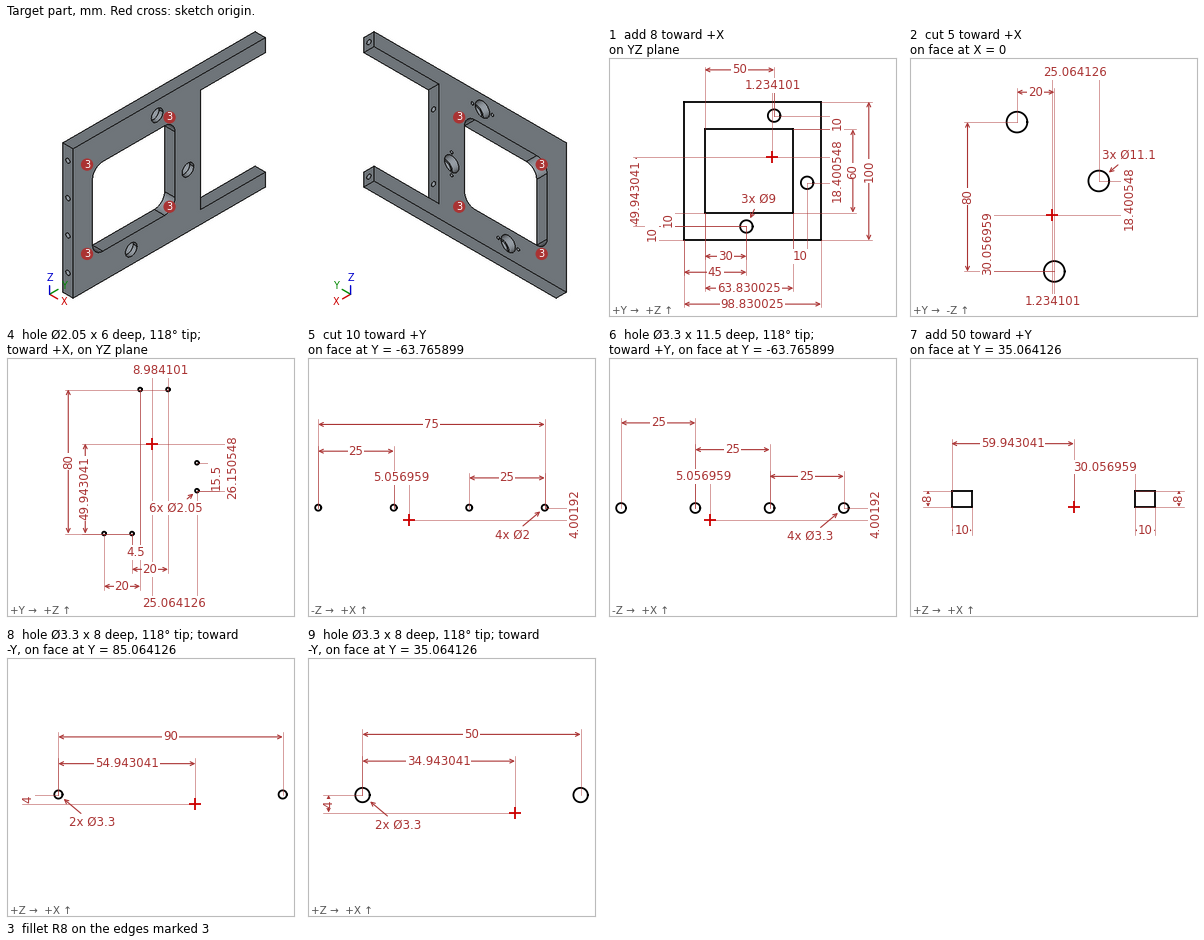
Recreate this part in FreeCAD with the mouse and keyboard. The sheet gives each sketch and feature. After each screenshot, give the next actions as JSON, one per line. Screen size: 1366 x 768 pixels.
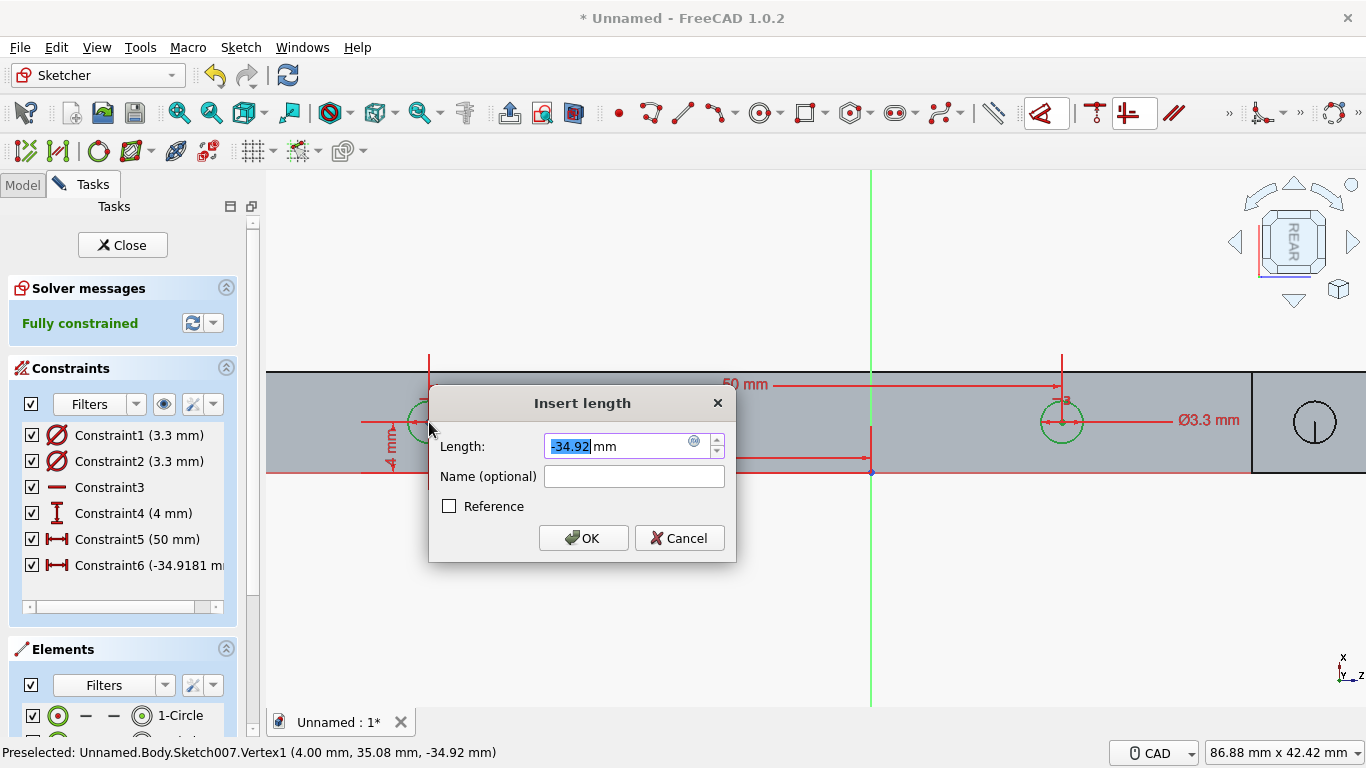
{"action": "type", "text": "-34.943041"}
{"action": "key", "text": "Return"}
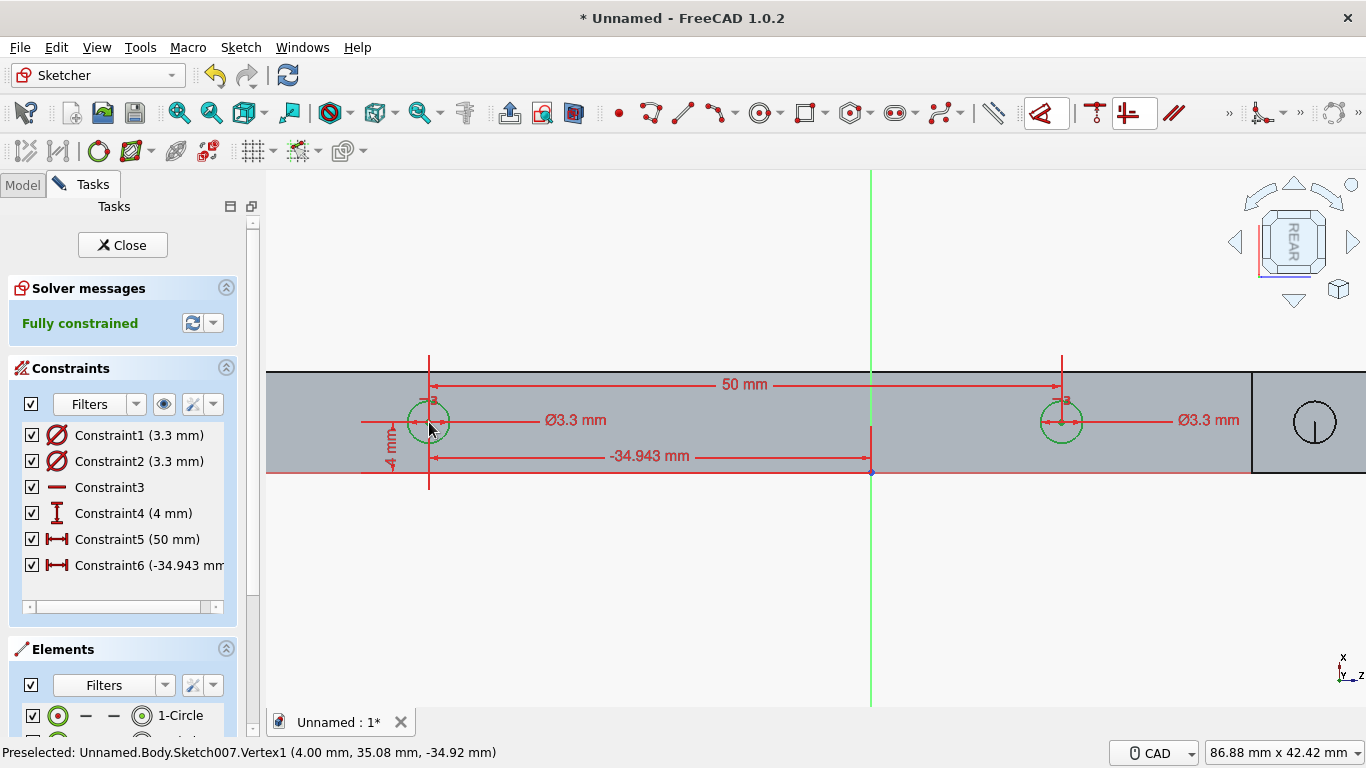
{"action": "left_click", "coordinate": [123, 245]}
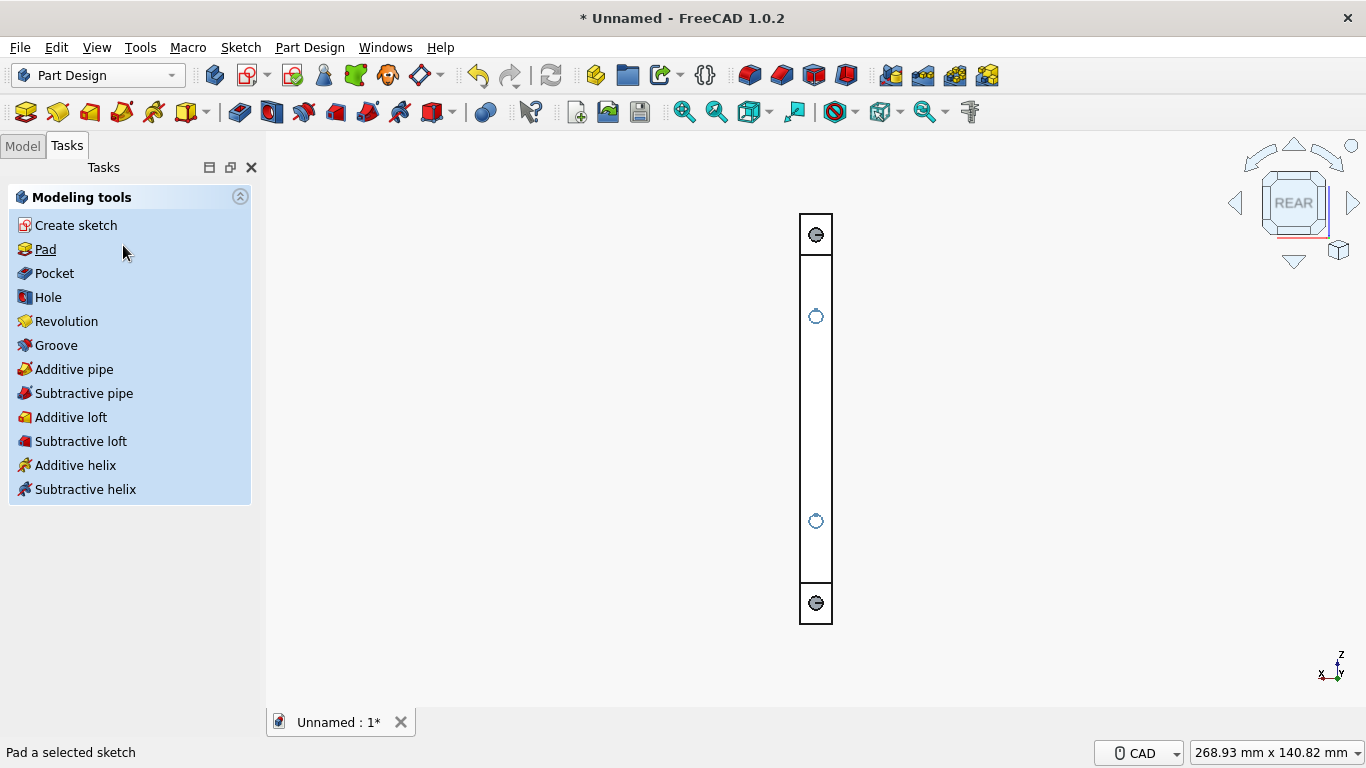
{"action": "left_click", "coordinate": [272, 112]}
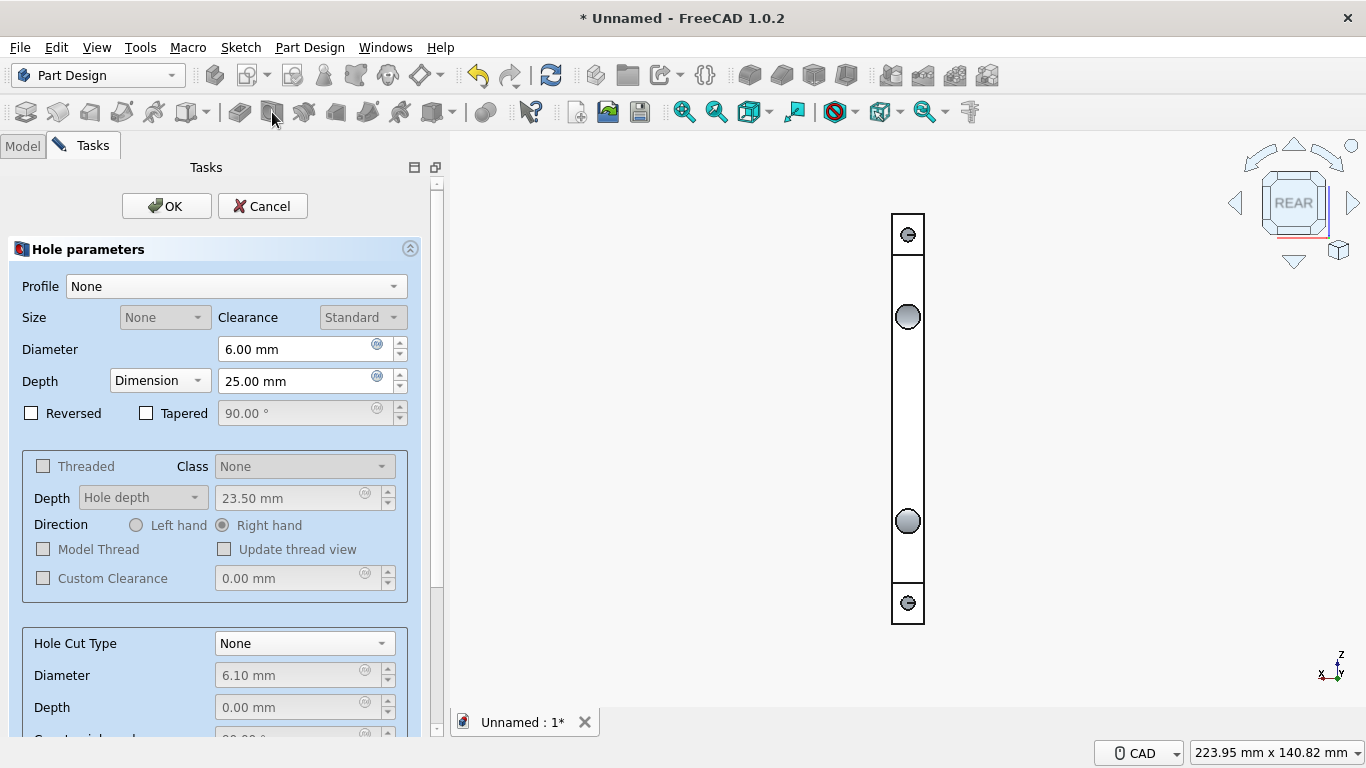
{"action": "triple_click", "coordinate": [305, 349]}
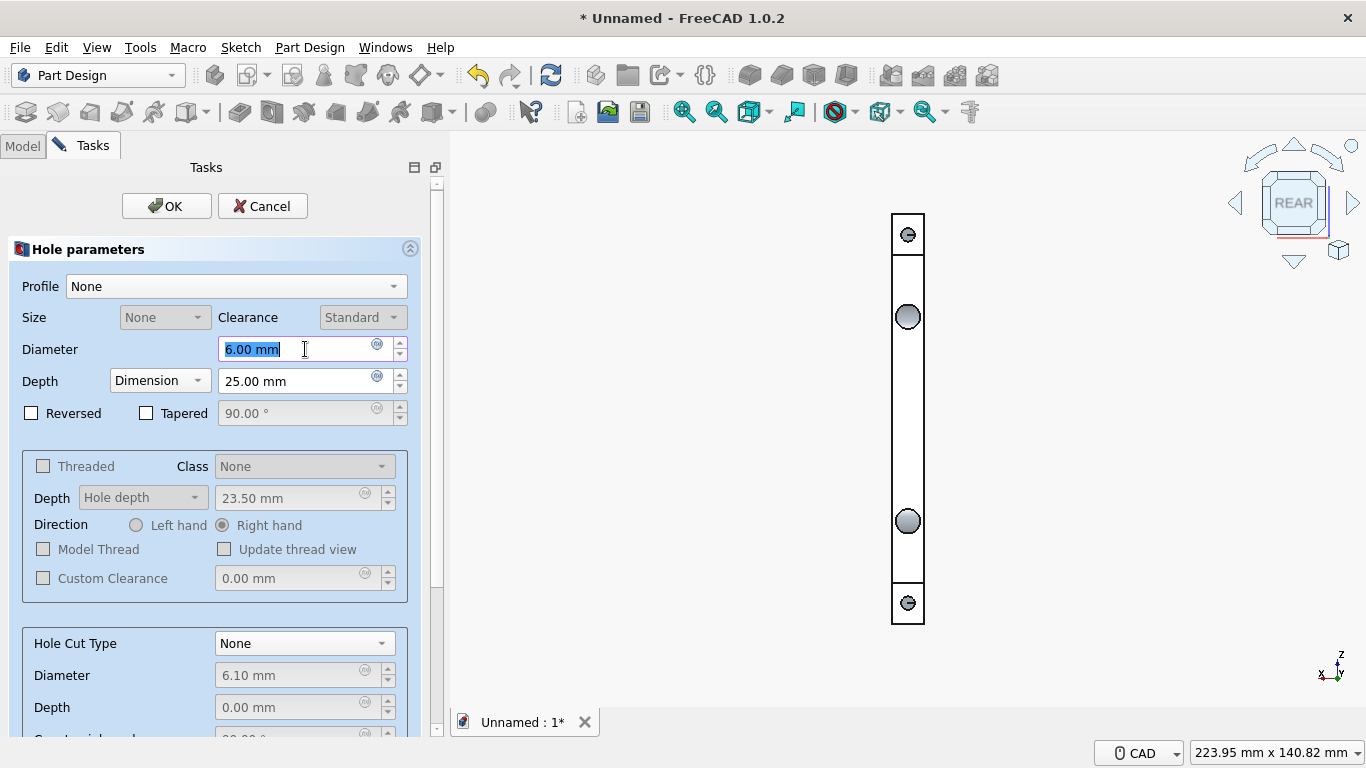
{"action": "type", "text": "3.3"}
{"action": "key", "text": "Tab"}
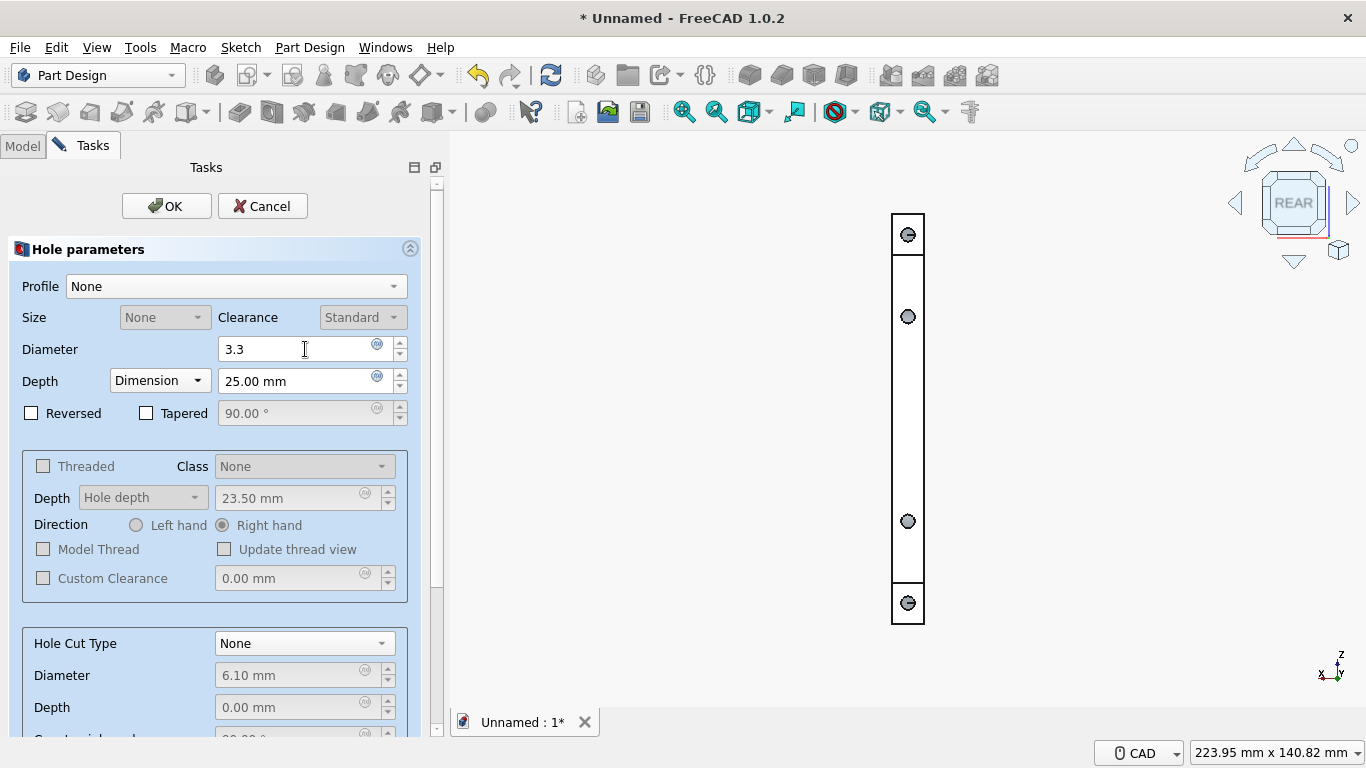
{"action": "triple_click", "coordinate": [305, 381]}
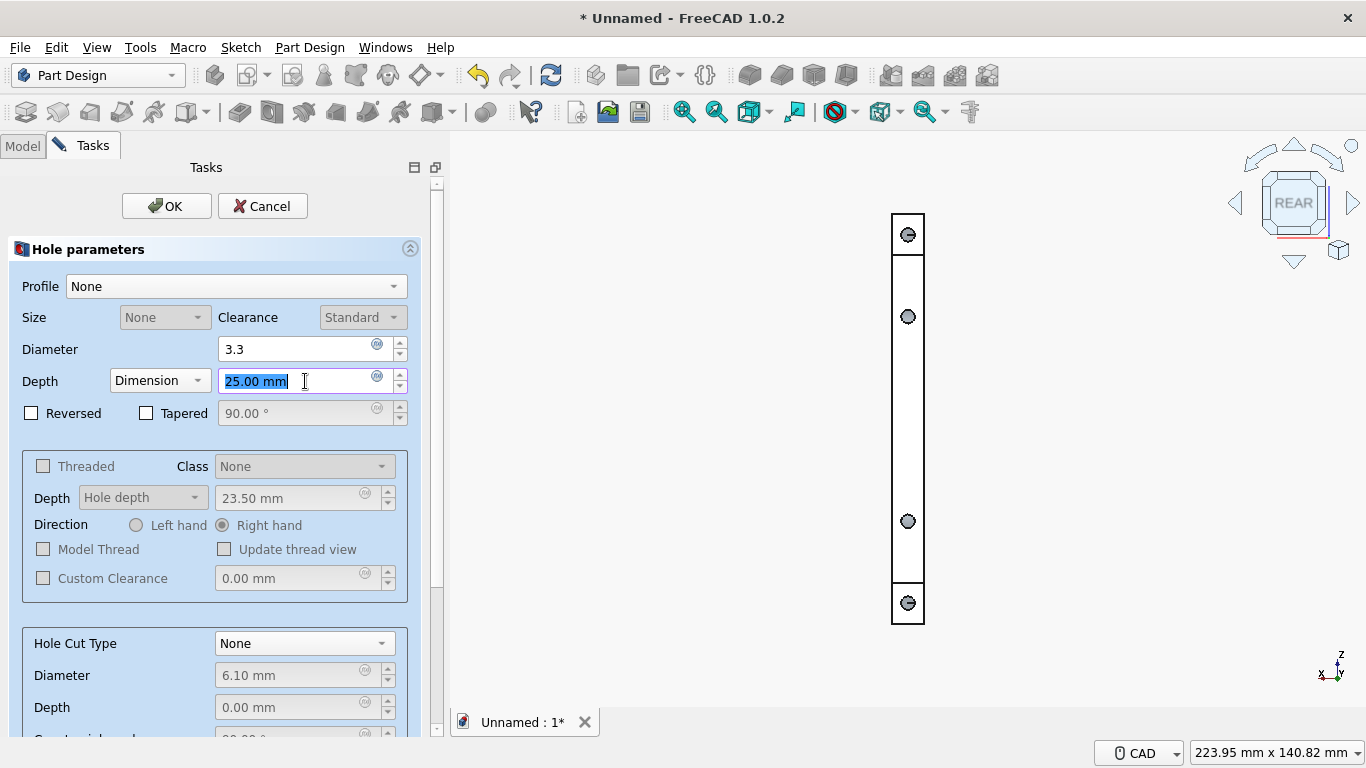
{"action": "type", "text": "8"}
{"action": "key", "text": "Tab"}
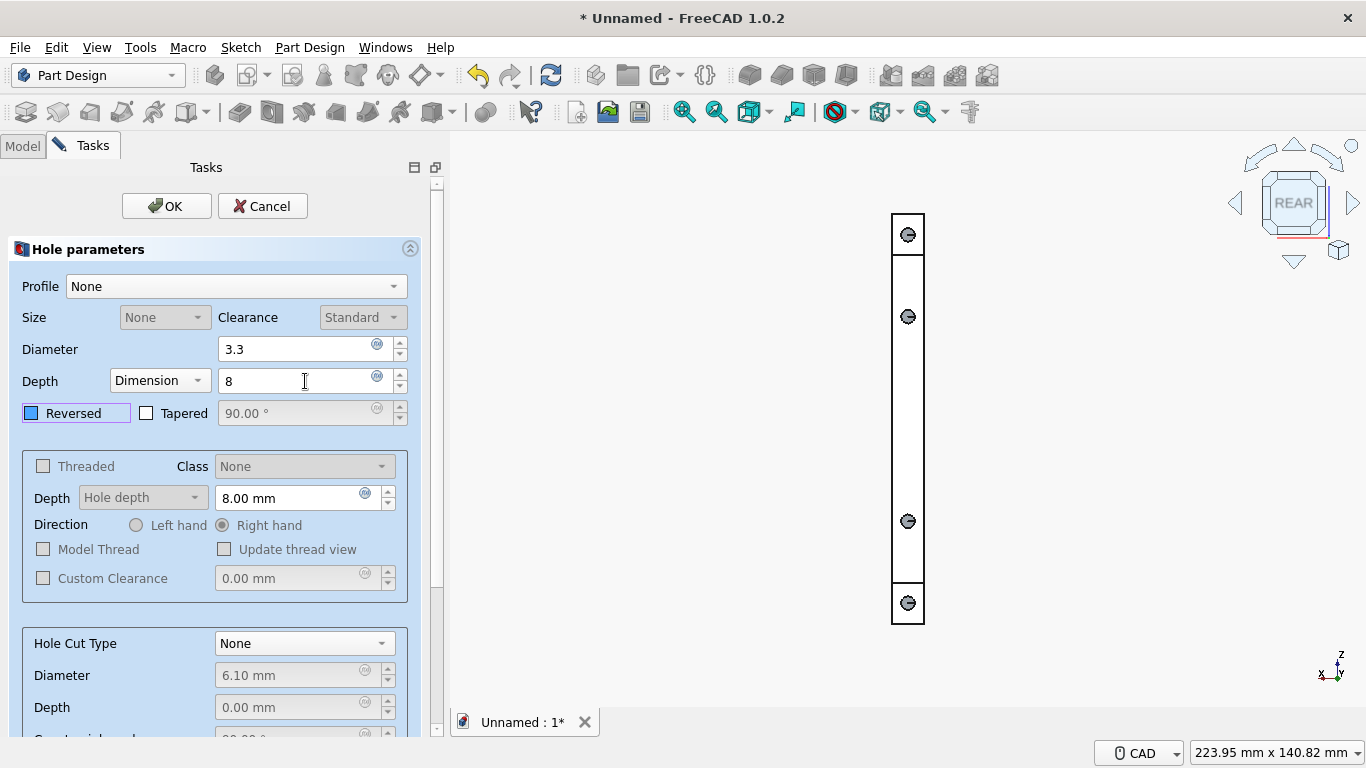
{"action": "left_click", "coordinate": [167, 206]}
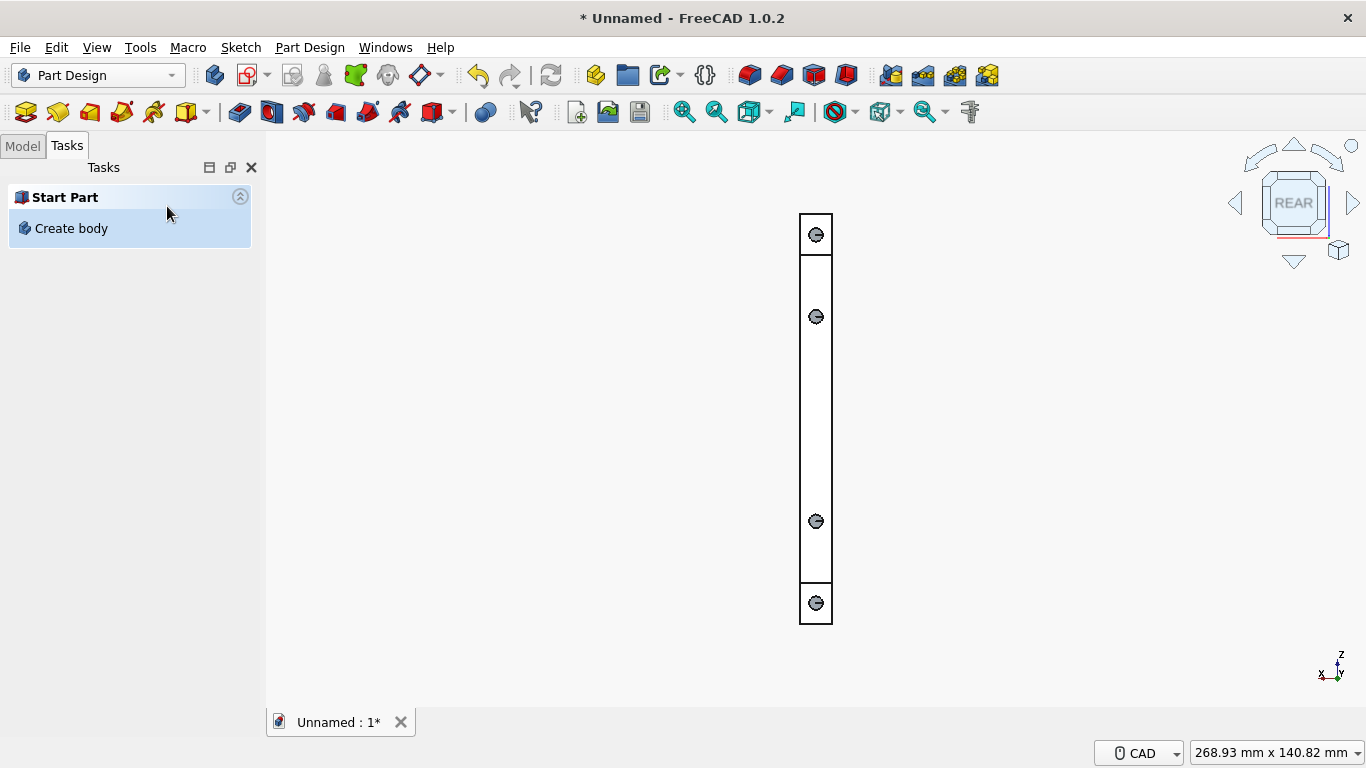
{"action": "key", "text": "0"}